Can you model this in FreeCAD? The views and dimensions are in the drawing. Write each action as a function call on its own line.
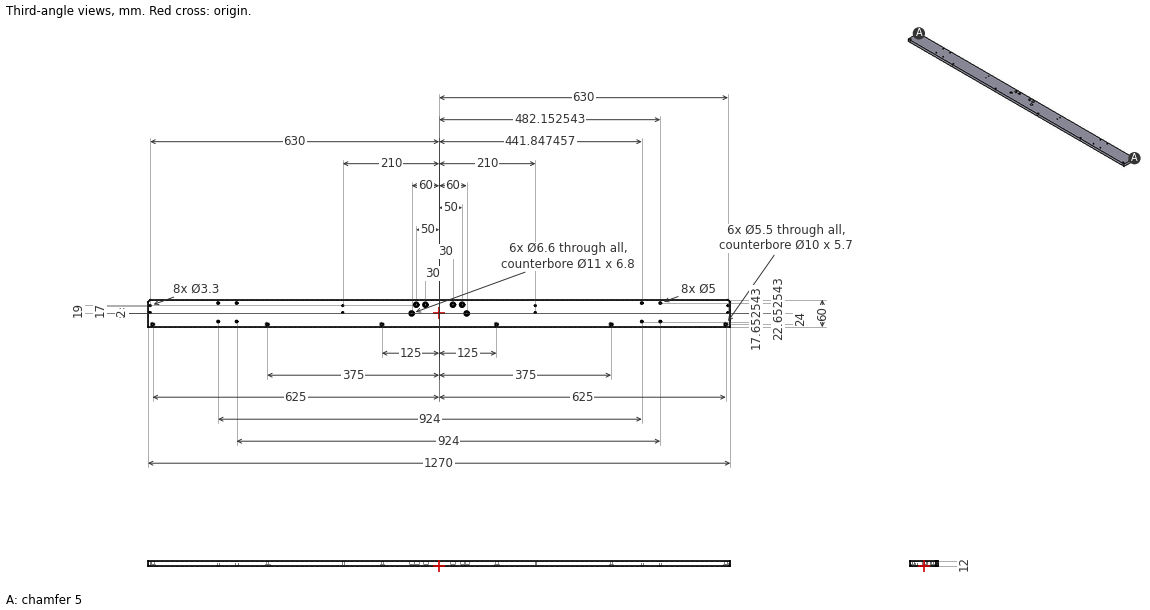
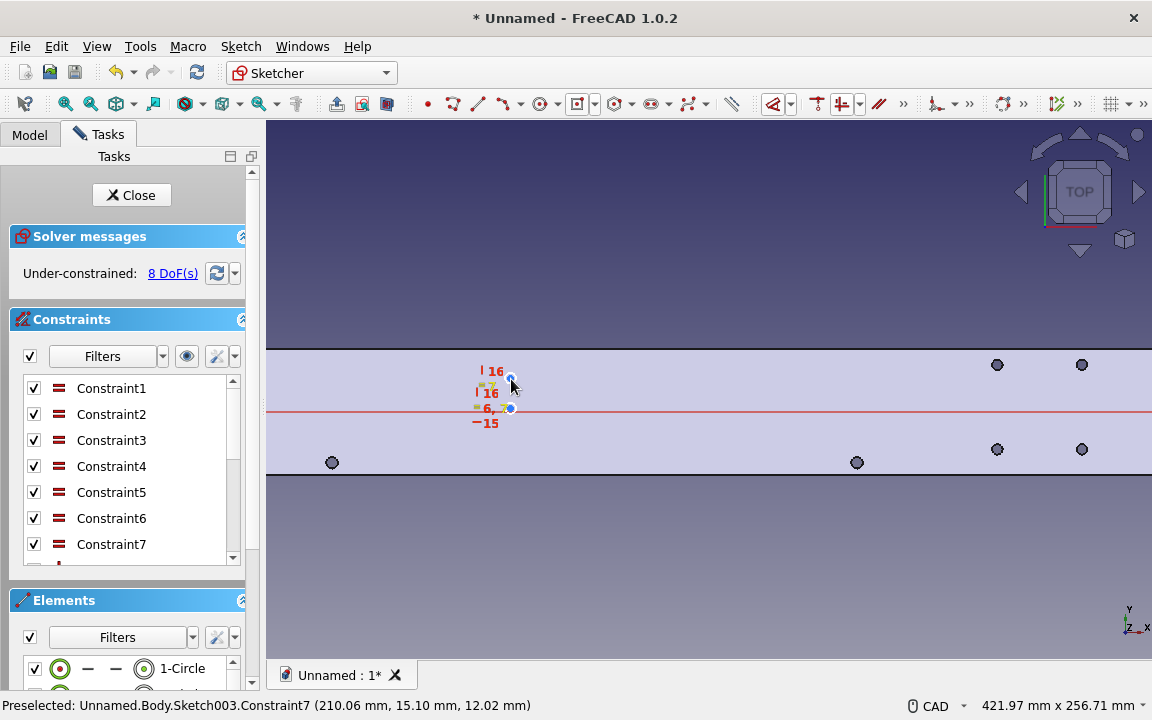
click(511, 378)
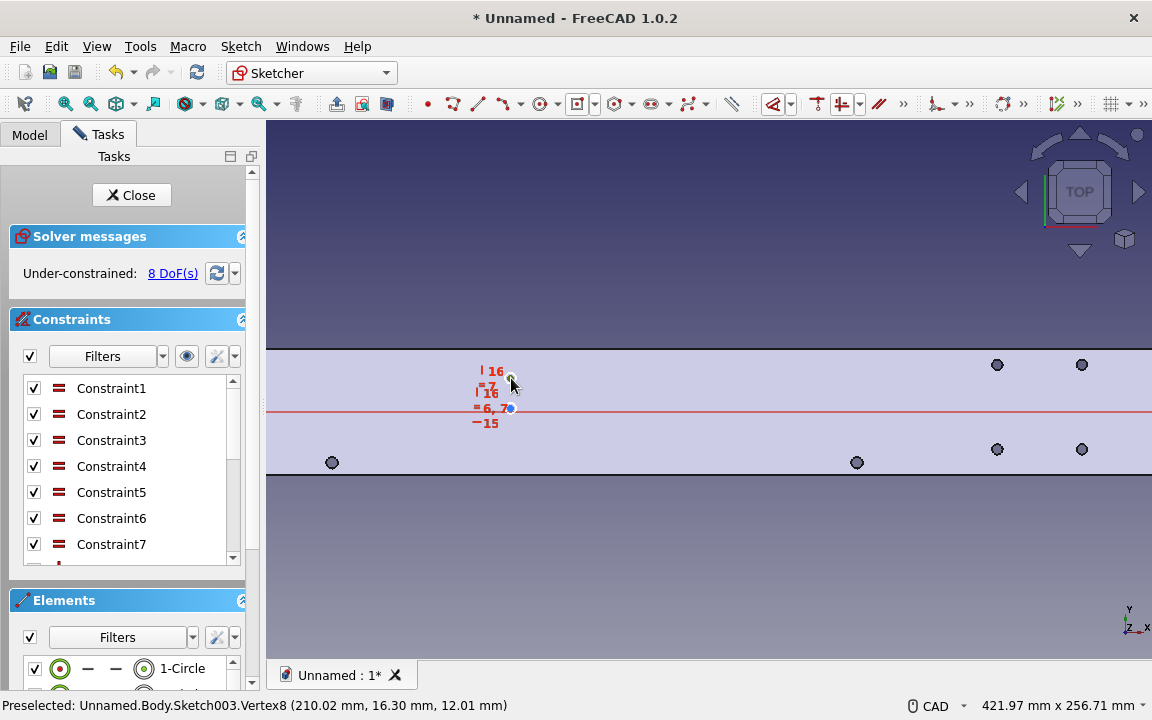
key(h)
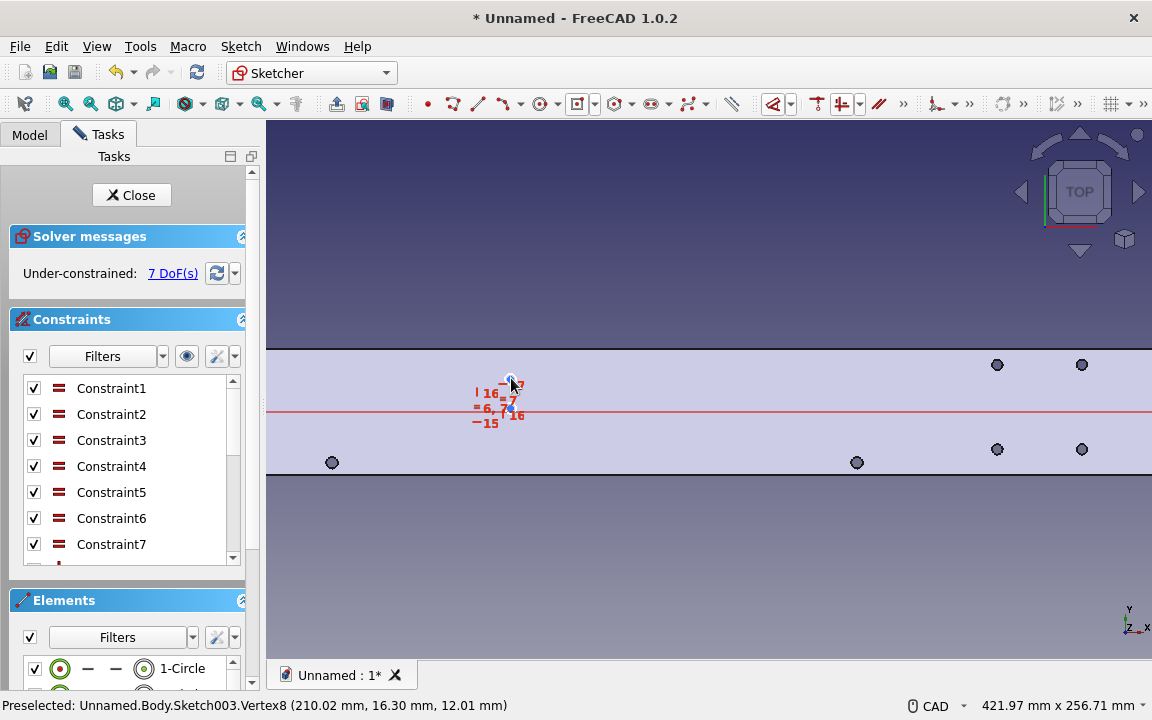
scroll(785, 389, down, 8)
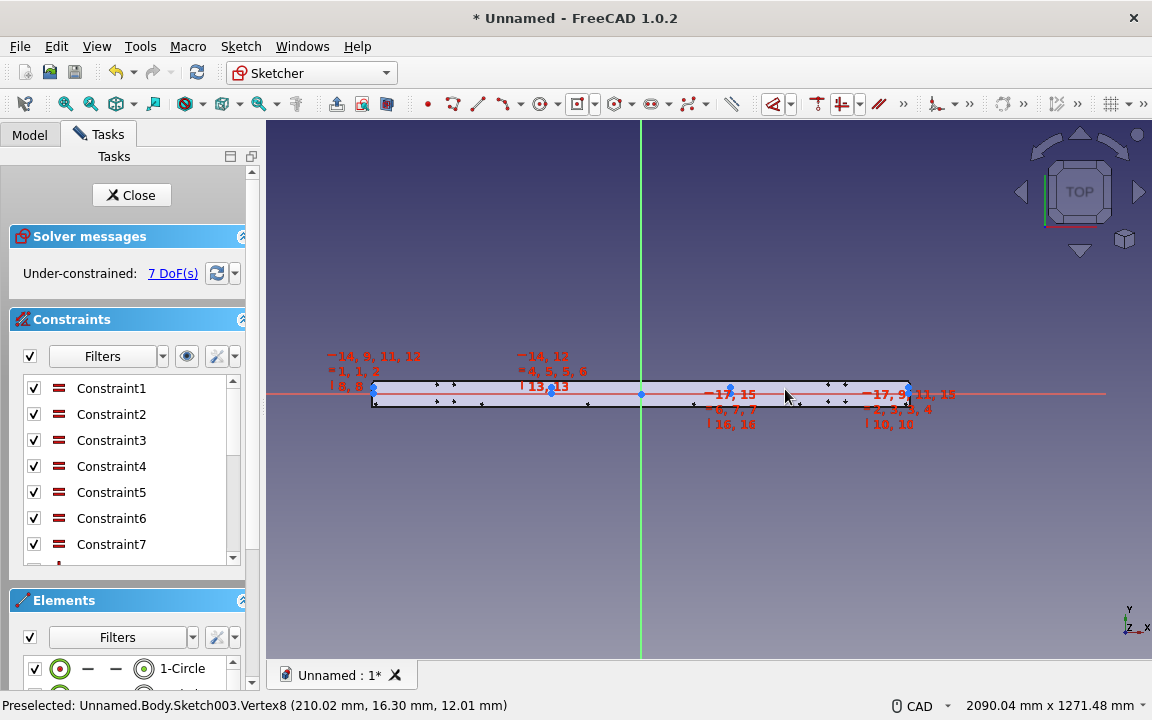
scroll(375, 387, up, 17)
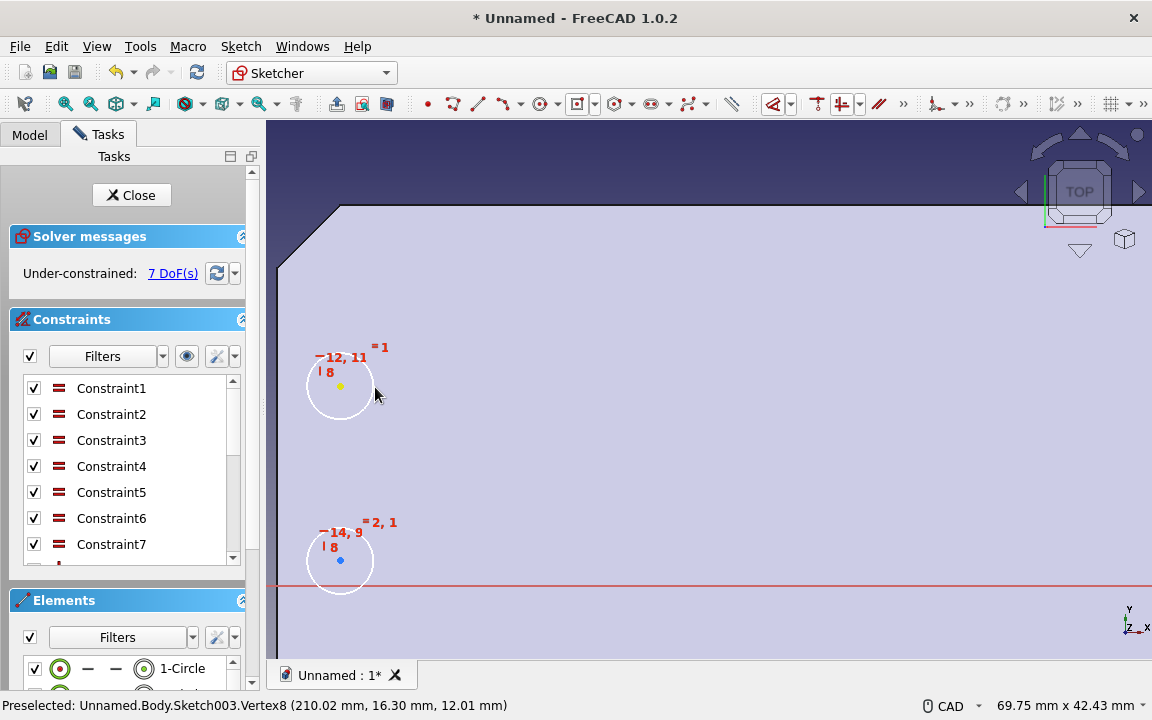
click(317, 410)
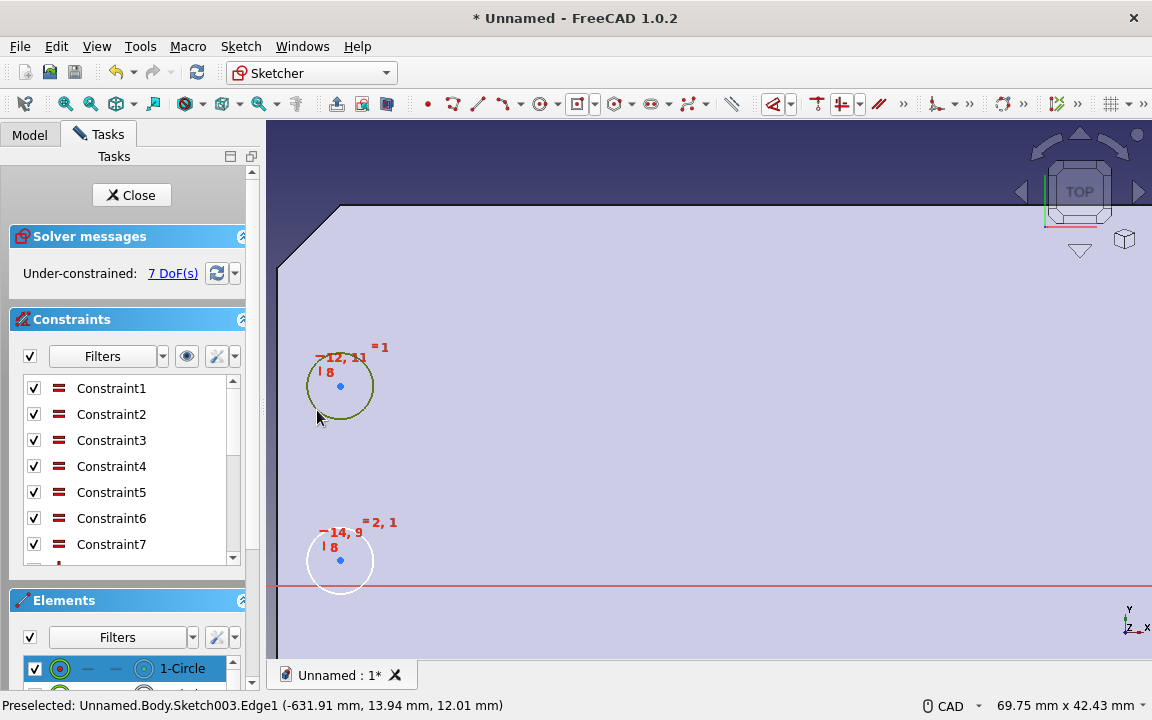
click(790, 104)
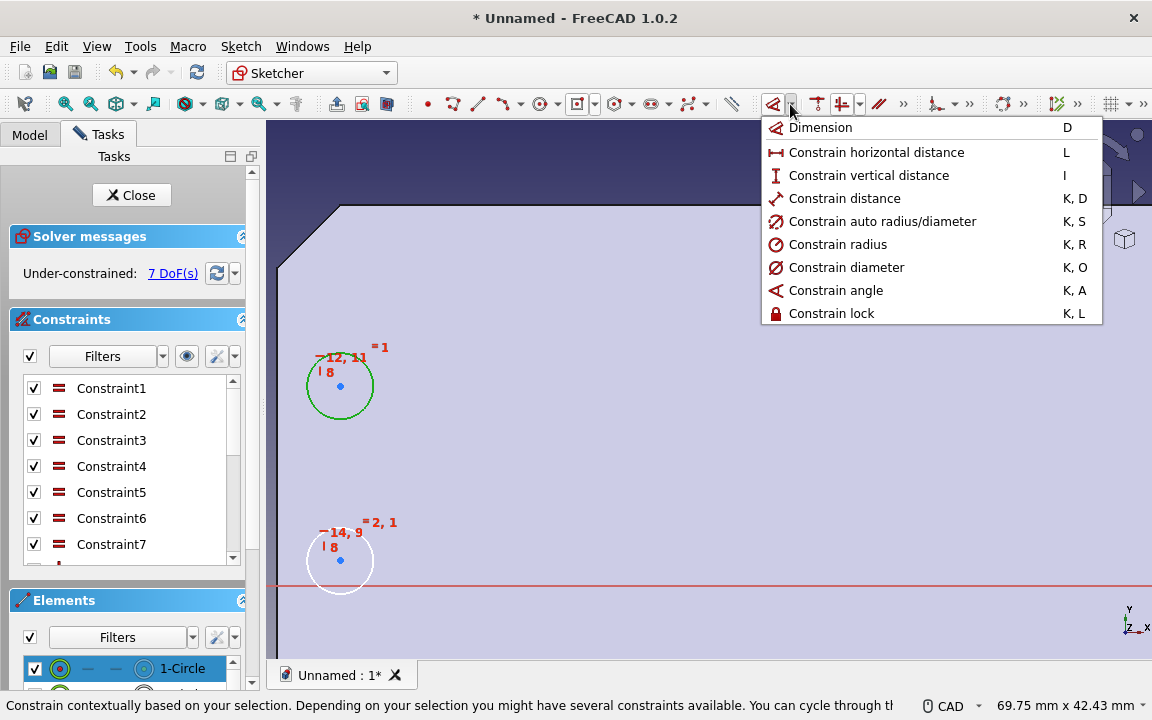
click(932, 268)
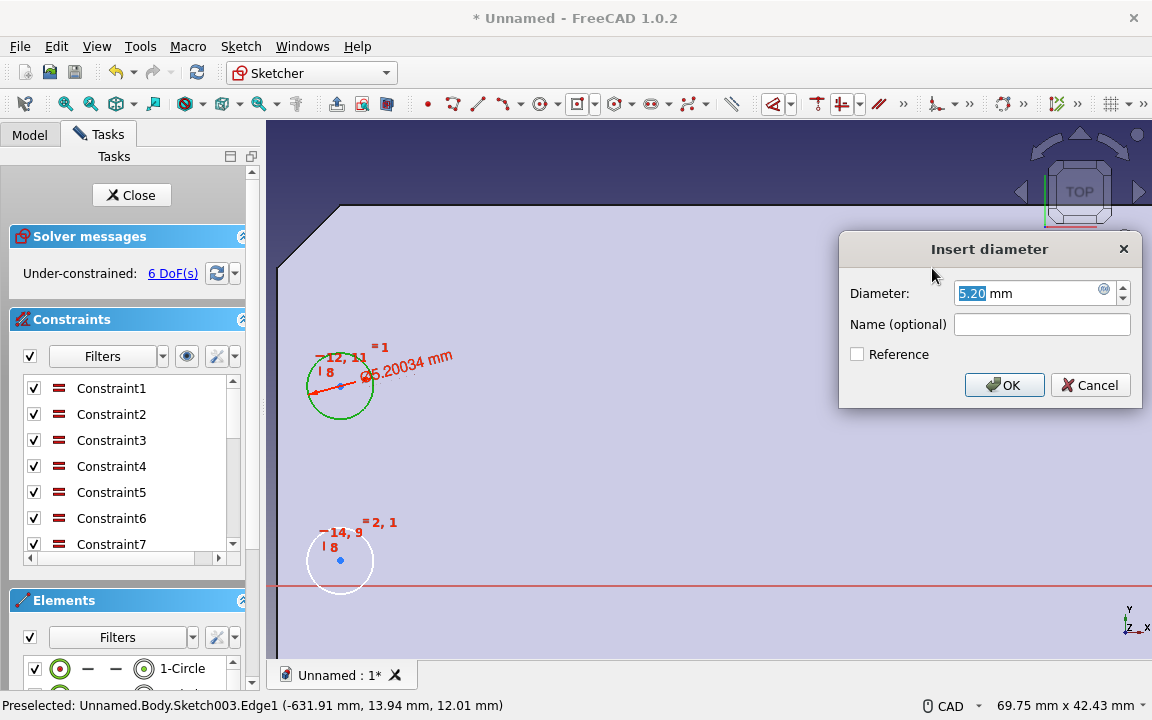
text(3.3)
key(Return)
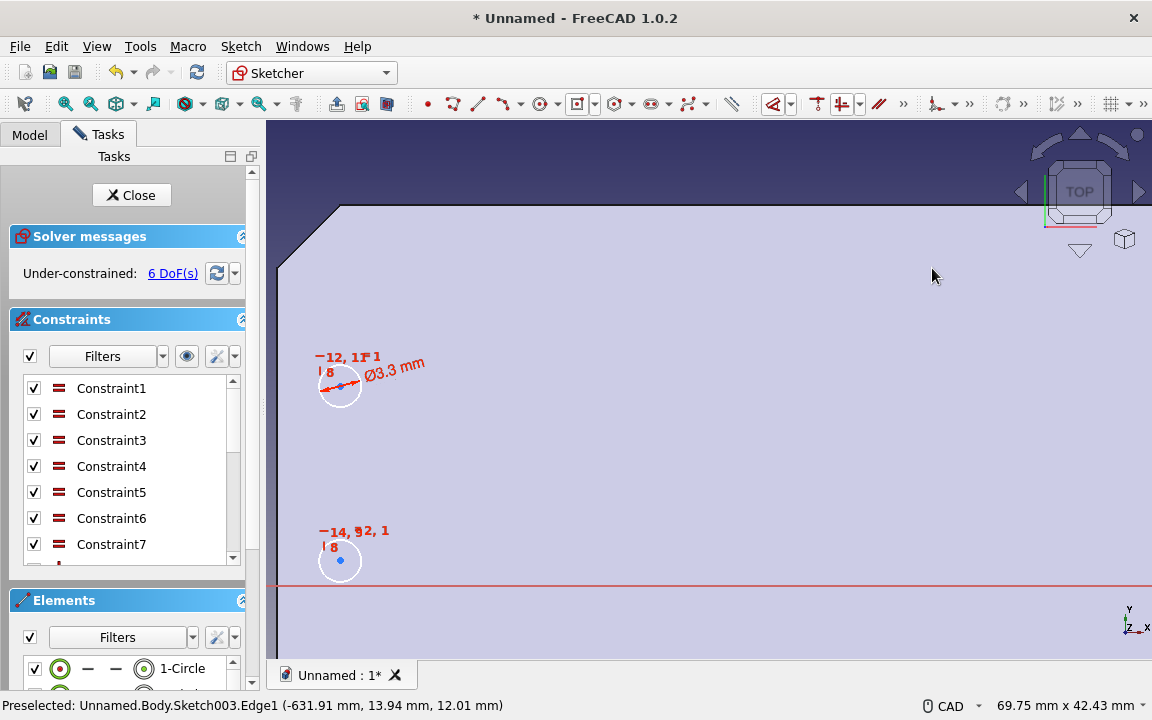
scroll(340, 561, up, 3)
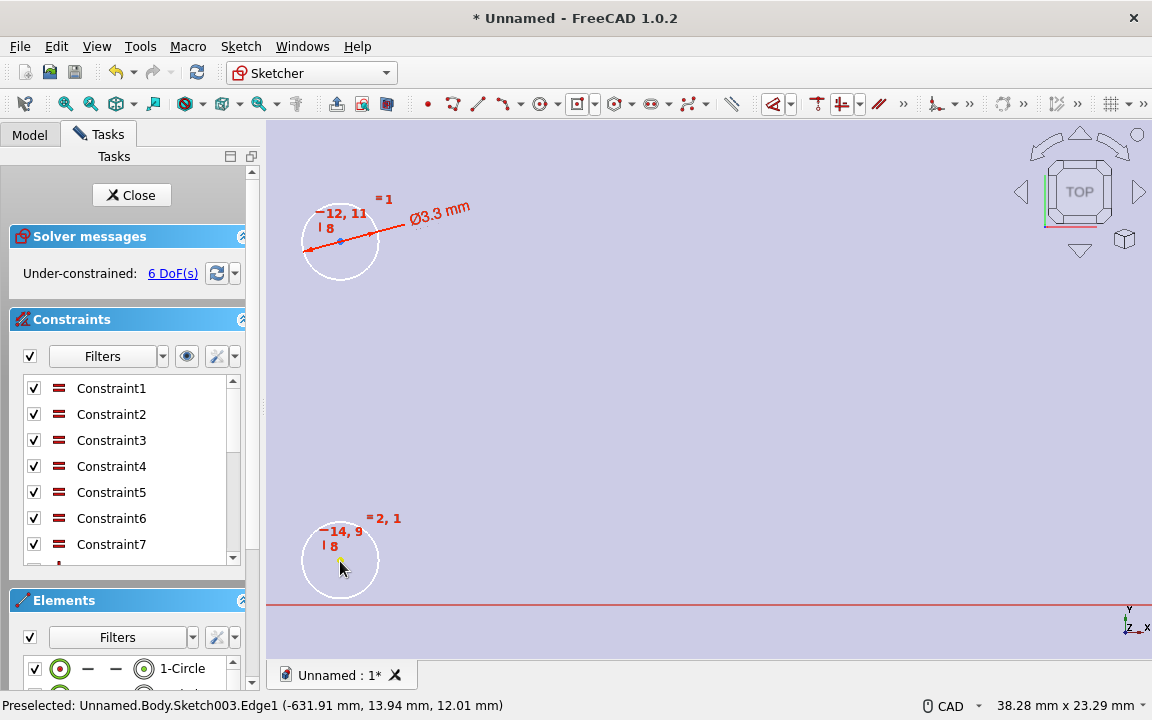
click(340, 560)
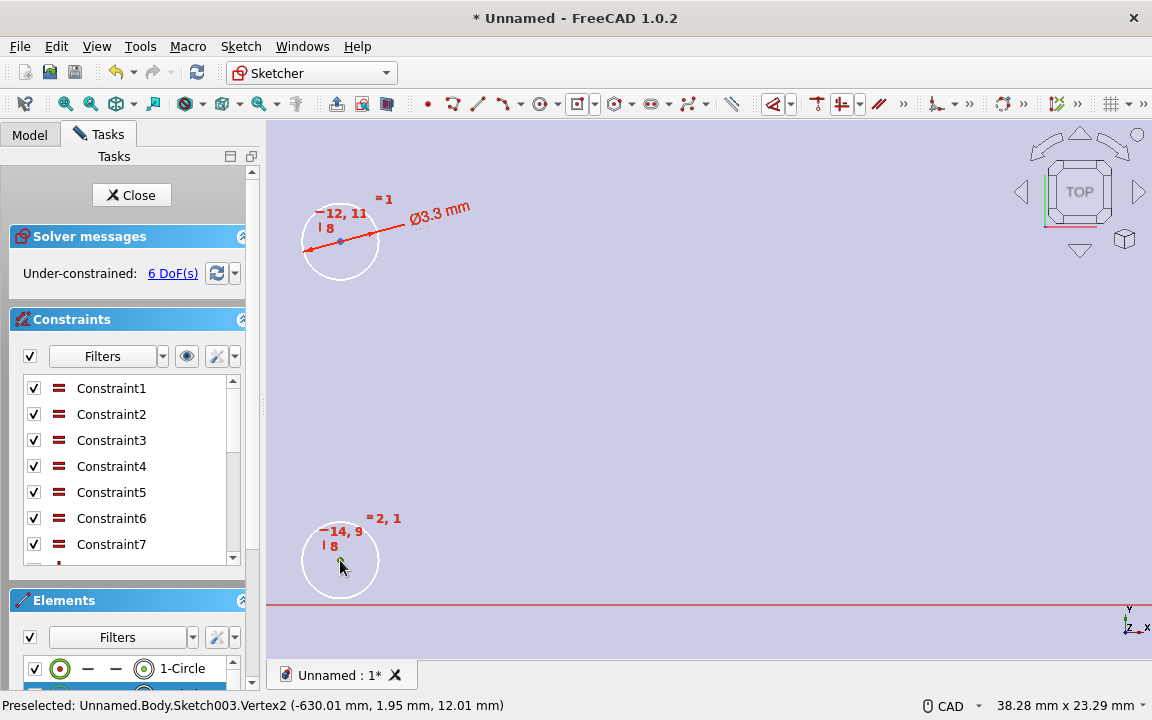
key(i)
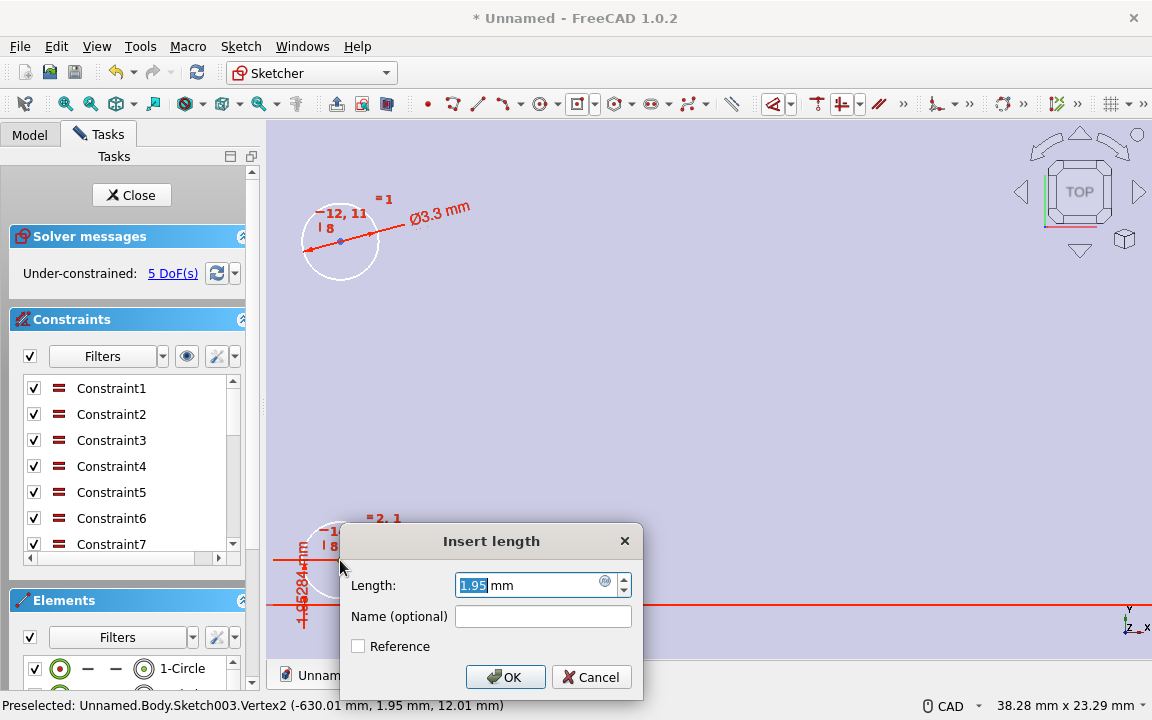
text(2)
key(Return)